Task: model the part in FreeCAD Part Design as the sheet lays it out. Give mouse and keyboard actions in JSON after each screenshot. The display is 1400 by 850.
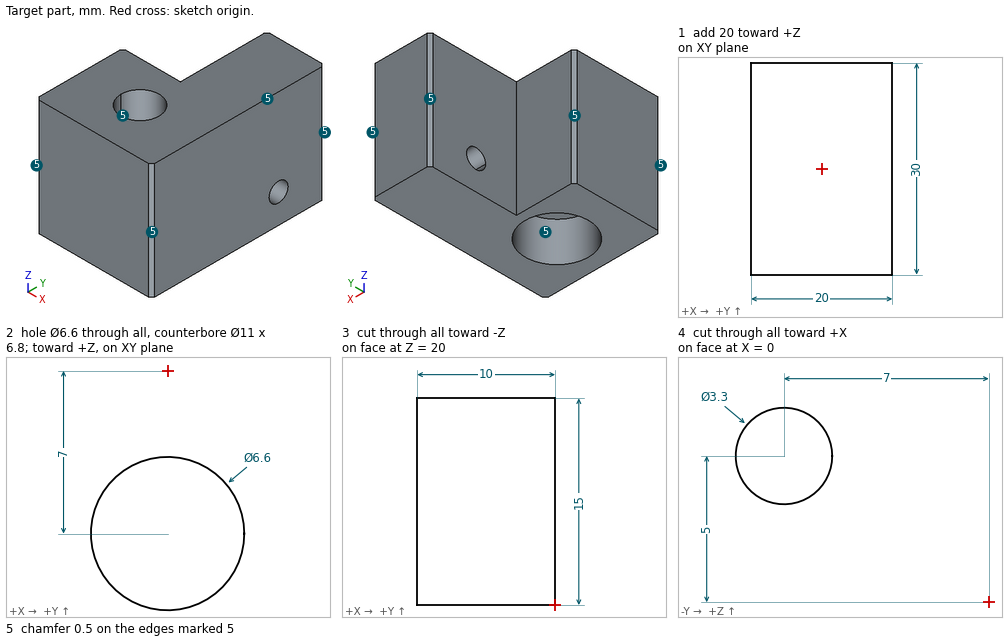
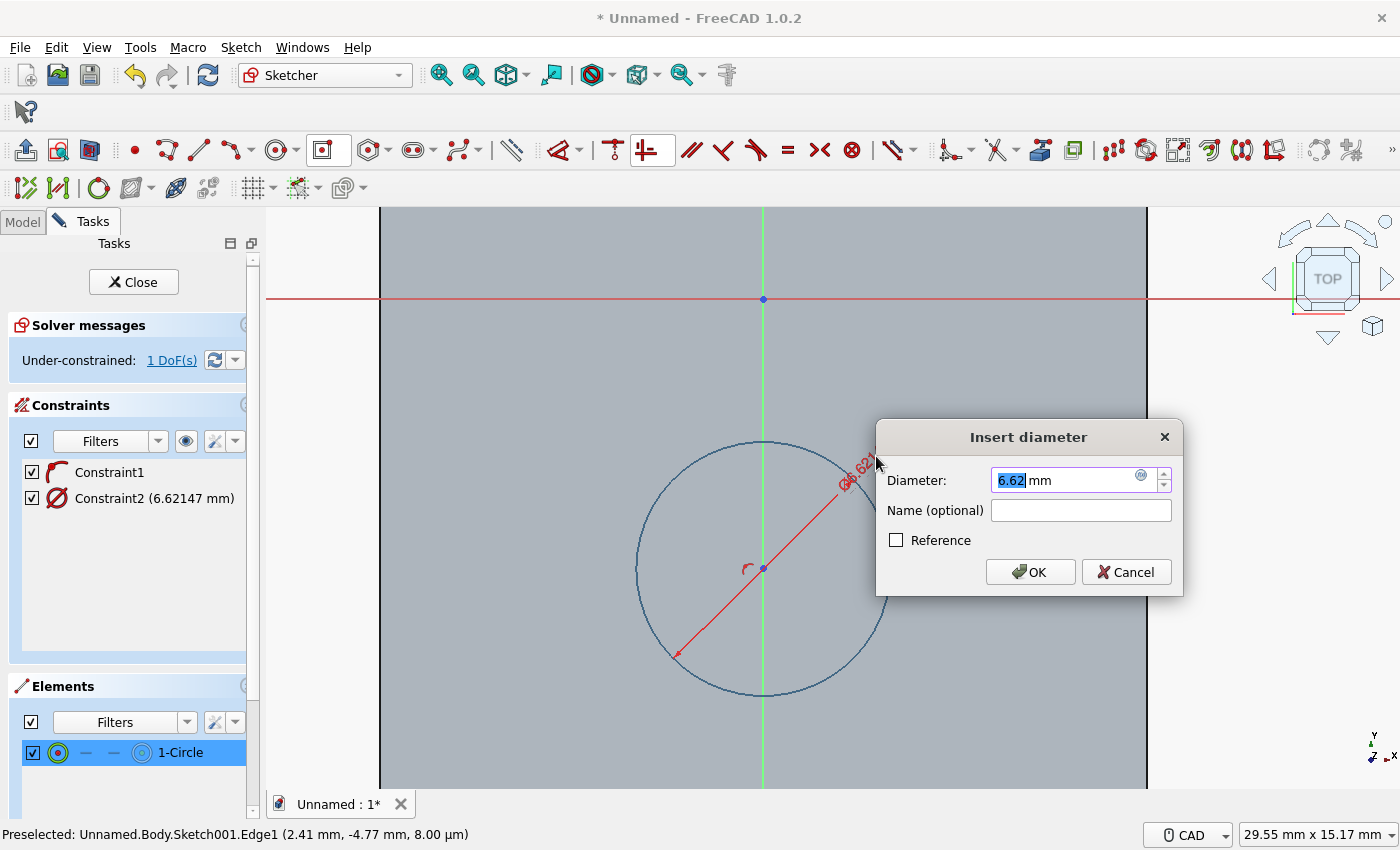
{"action": "type", "text": "6.6"}
{"action": "key", "text": "Return"}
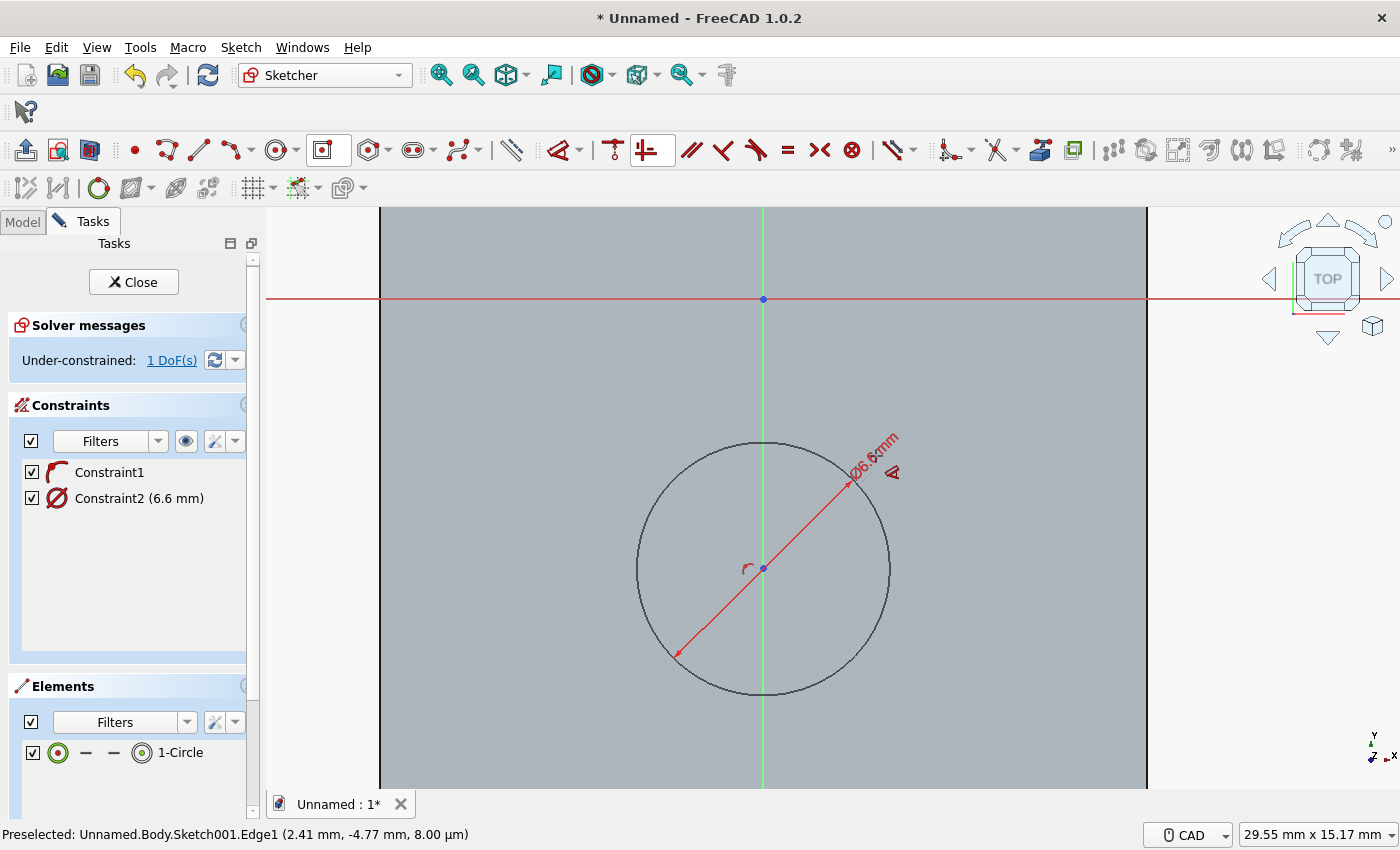
{"action": "left_click", "coordinate": [763, 569]}
{"action": "left_click", "coordinate": [797, 372]}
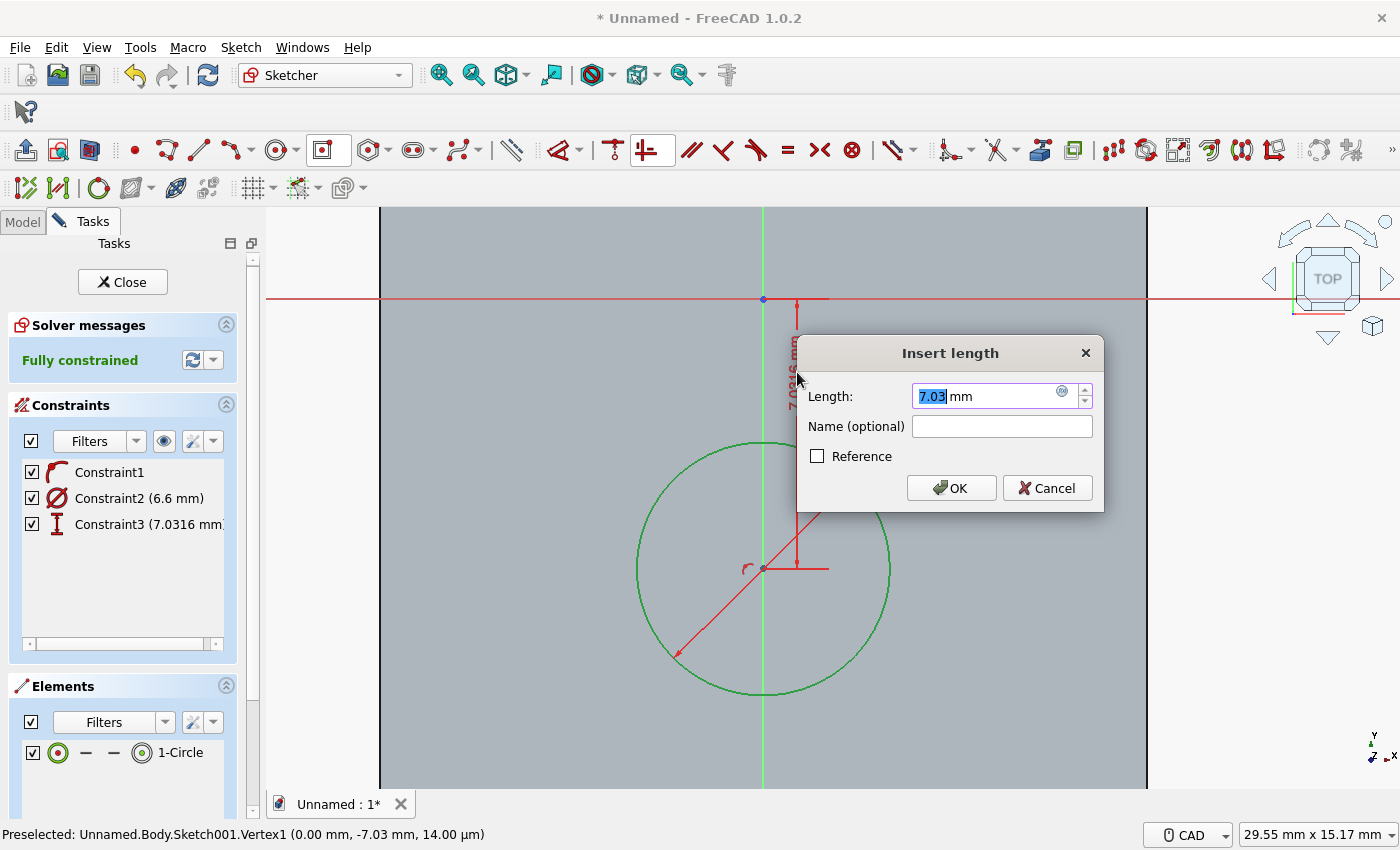
{"action": "type", "text": "7"}
{"action": "key", "text": "Return"}
{"action": "key", "text": "Escape"}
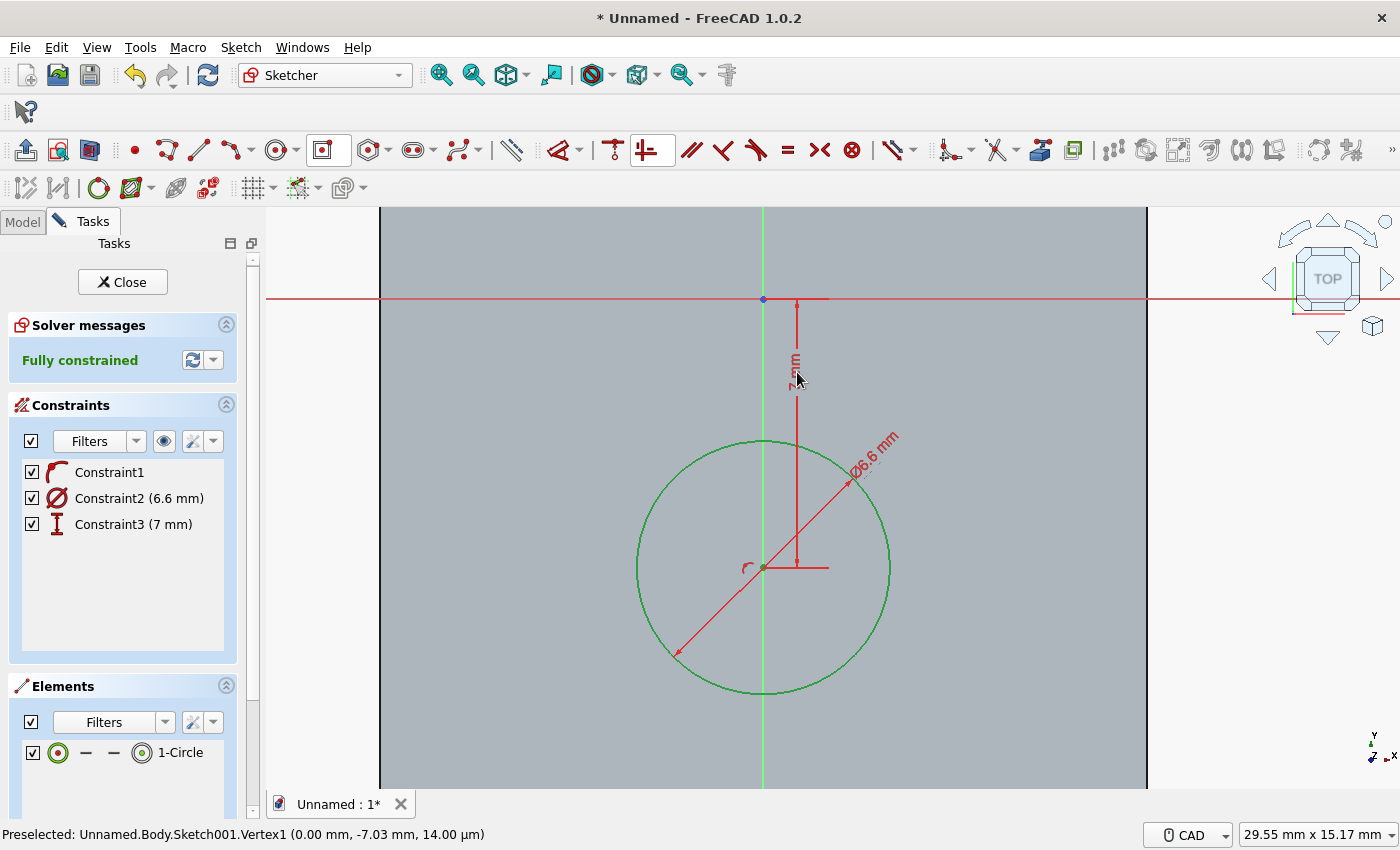
{"action": "left_click", "coordinate": [123, 282]}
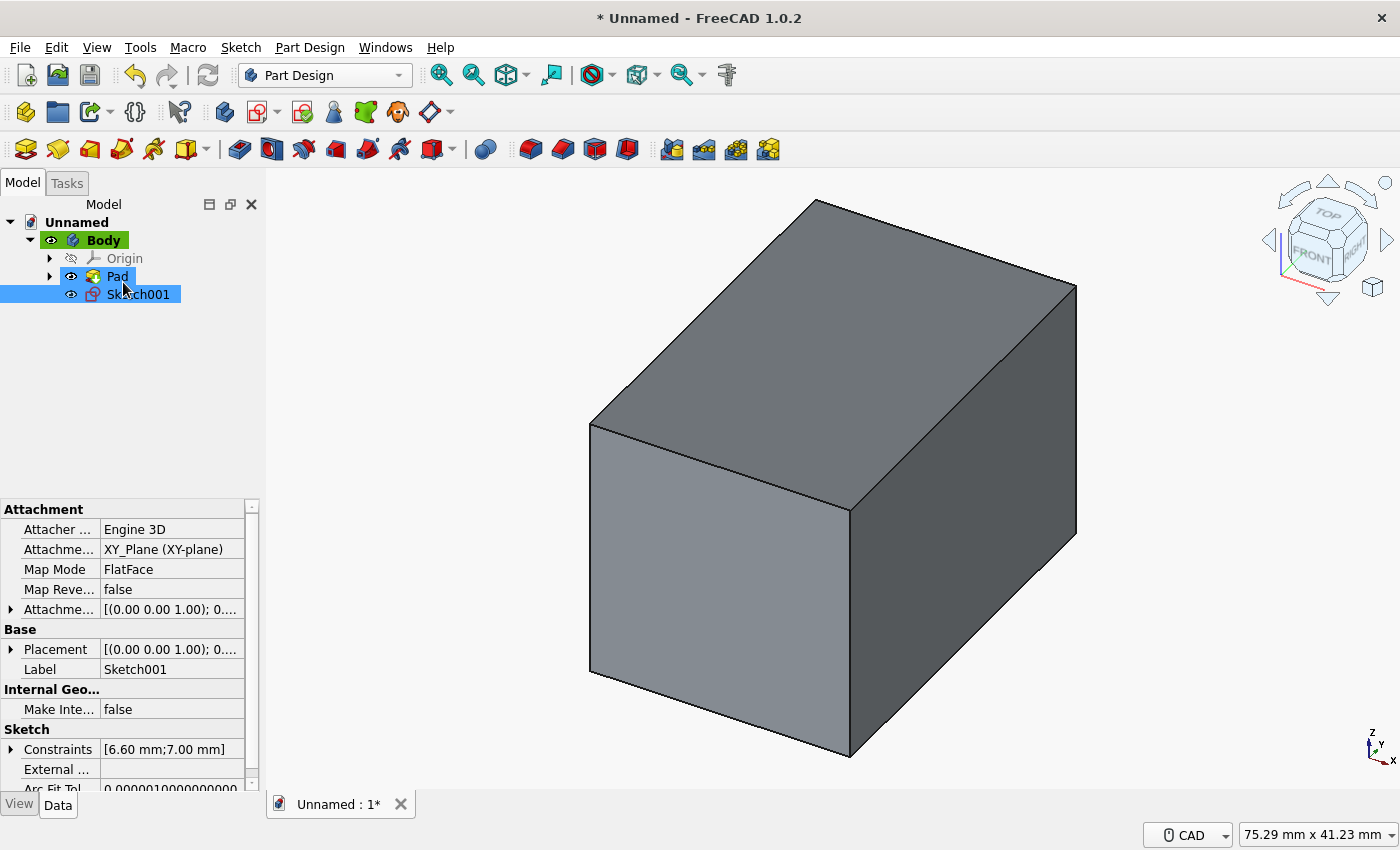
{"action": "left_click", "coordinate": [272, 150]}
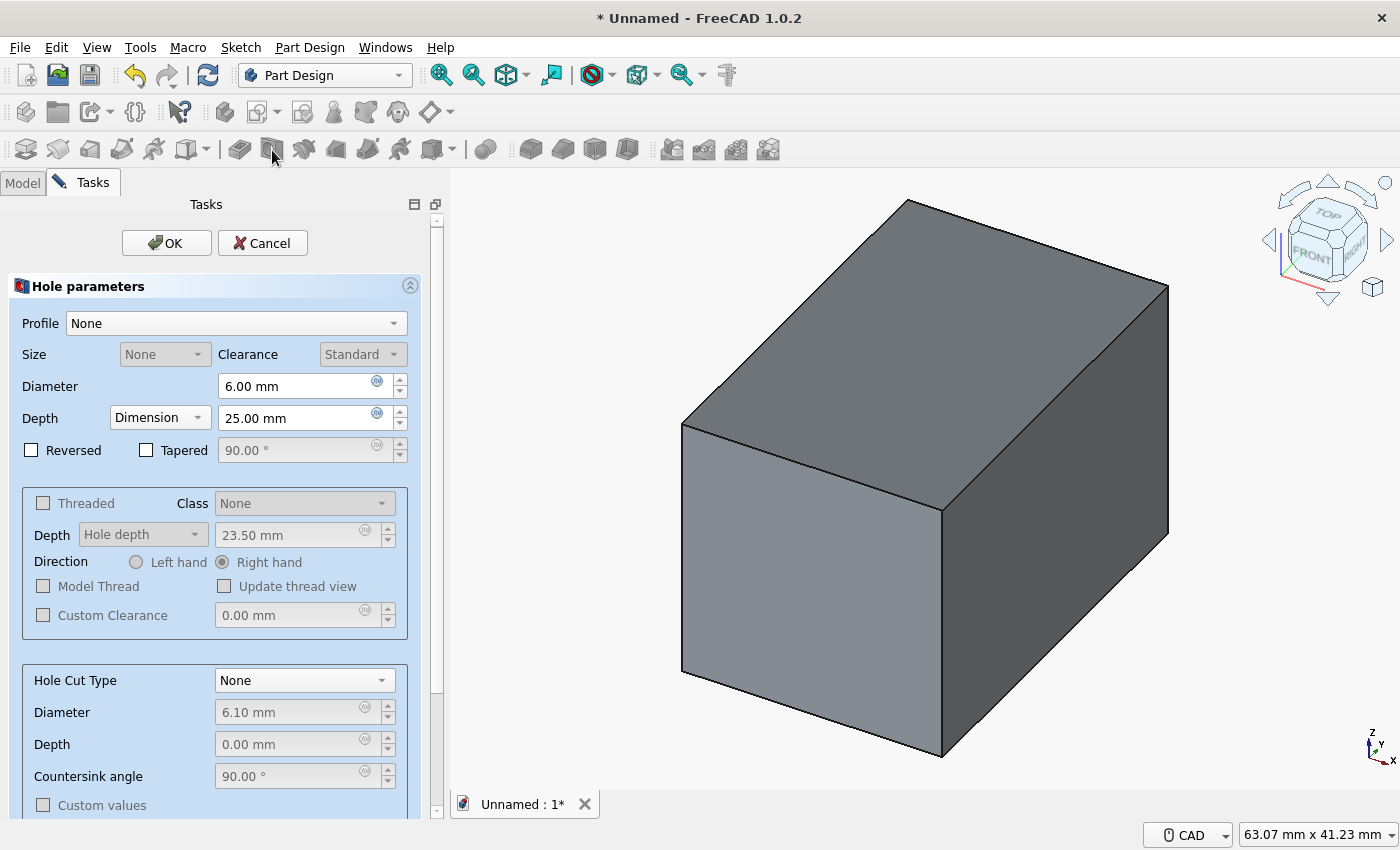
{"action": "triple_click", "coordinate": [305, 386]}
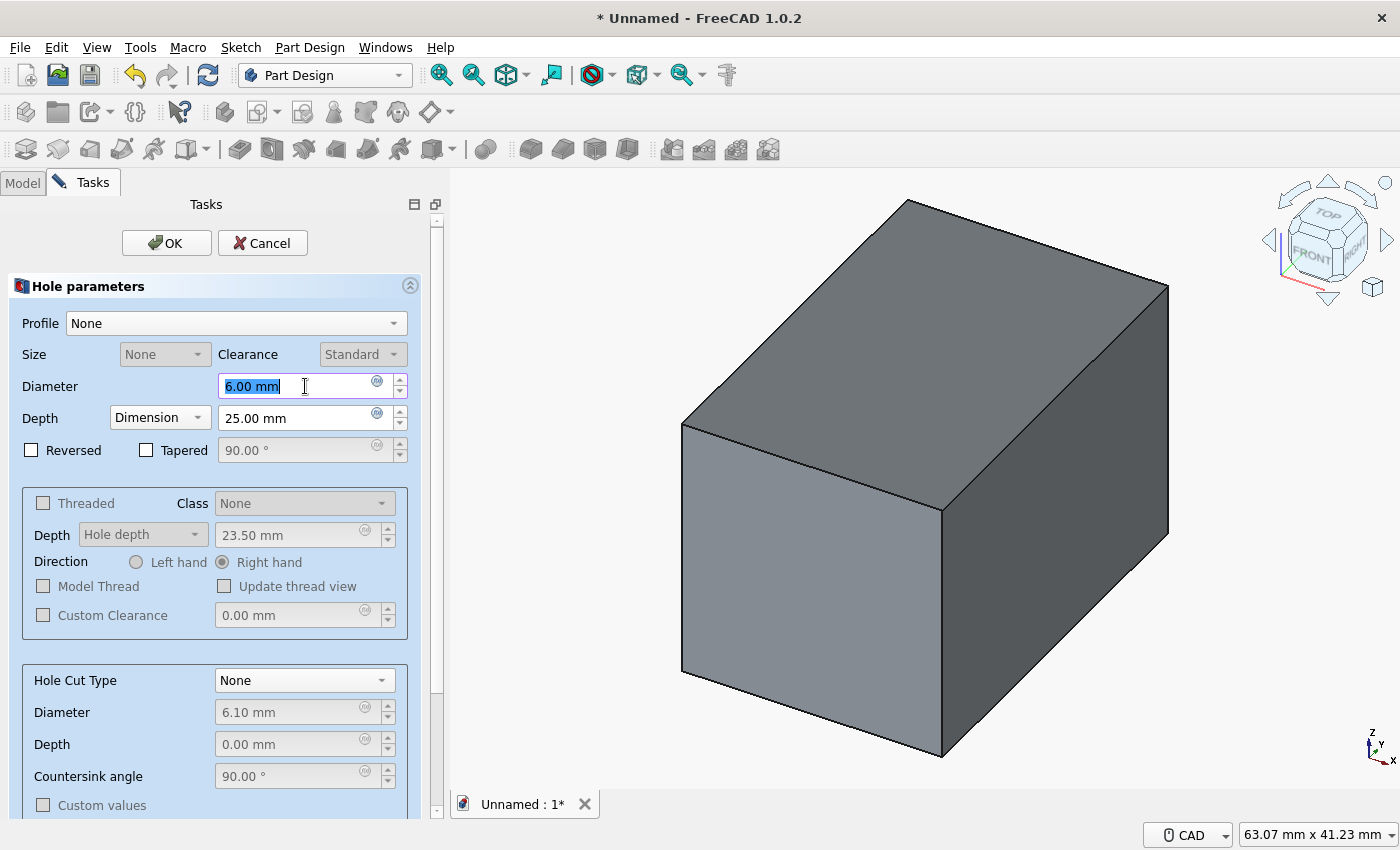
{"action": "type", "text": "6.6"}
{"action": "key", "text": "Tab"}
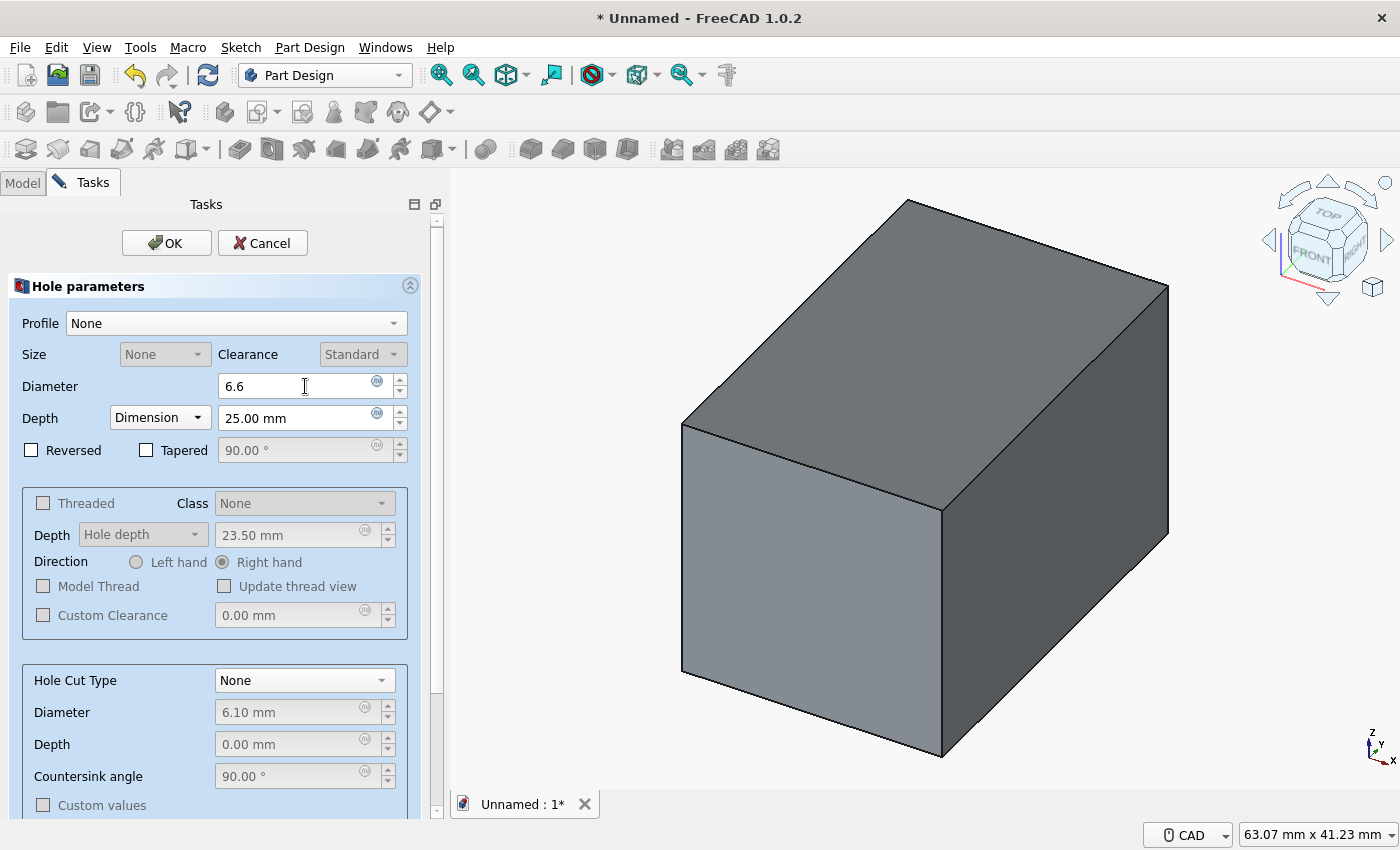
{"action": "left_click", "coordinate": [161, 418]}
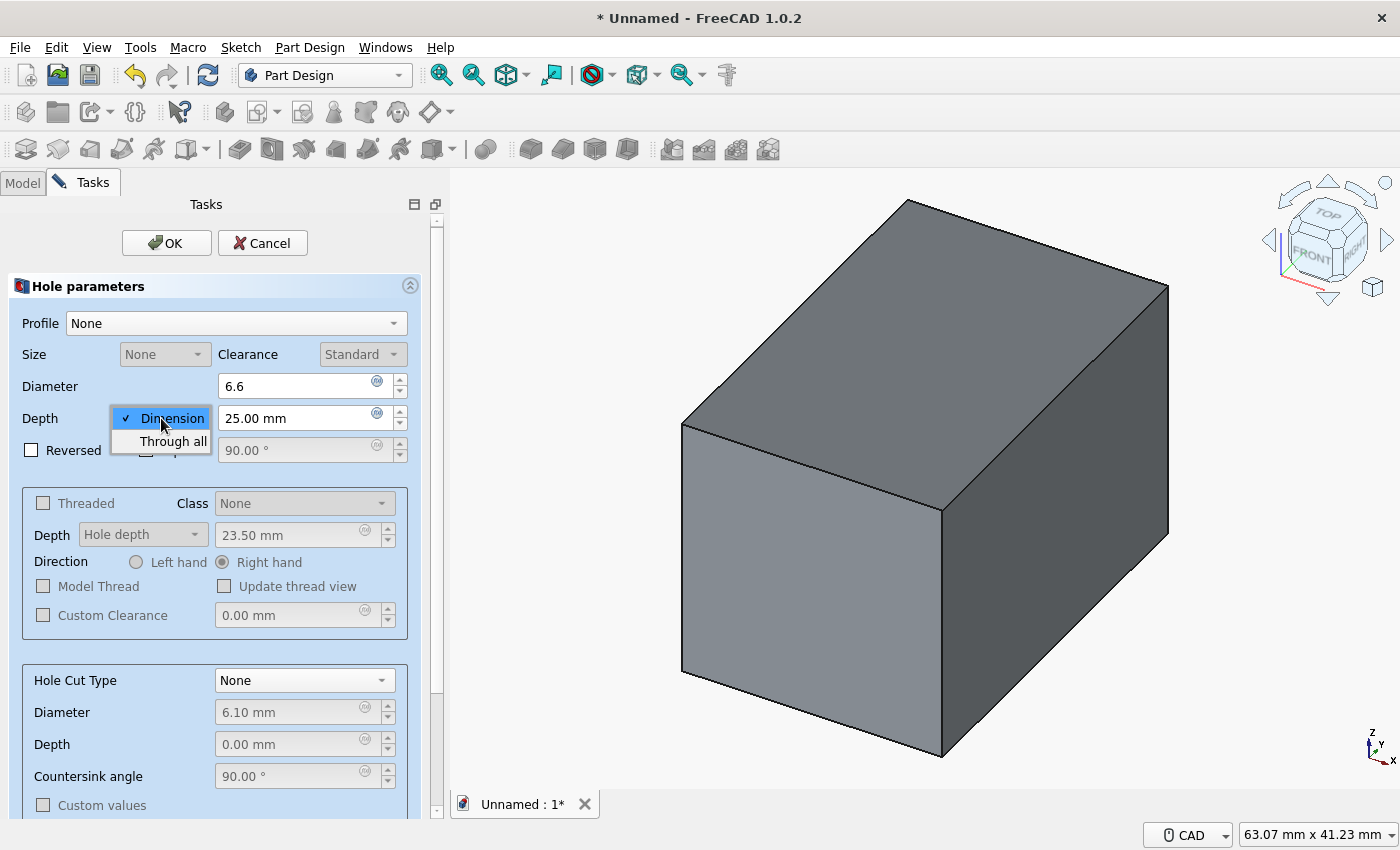
{"action": "left_click", "coordinate": [160, 442]}